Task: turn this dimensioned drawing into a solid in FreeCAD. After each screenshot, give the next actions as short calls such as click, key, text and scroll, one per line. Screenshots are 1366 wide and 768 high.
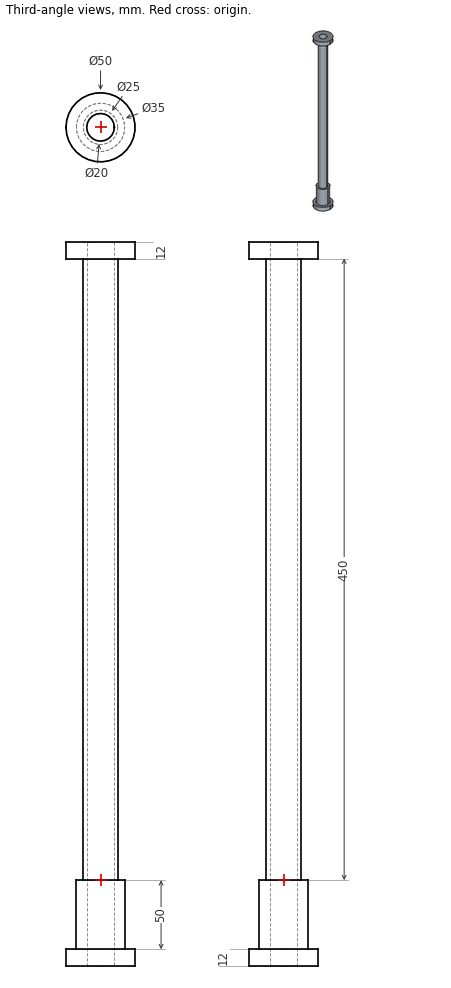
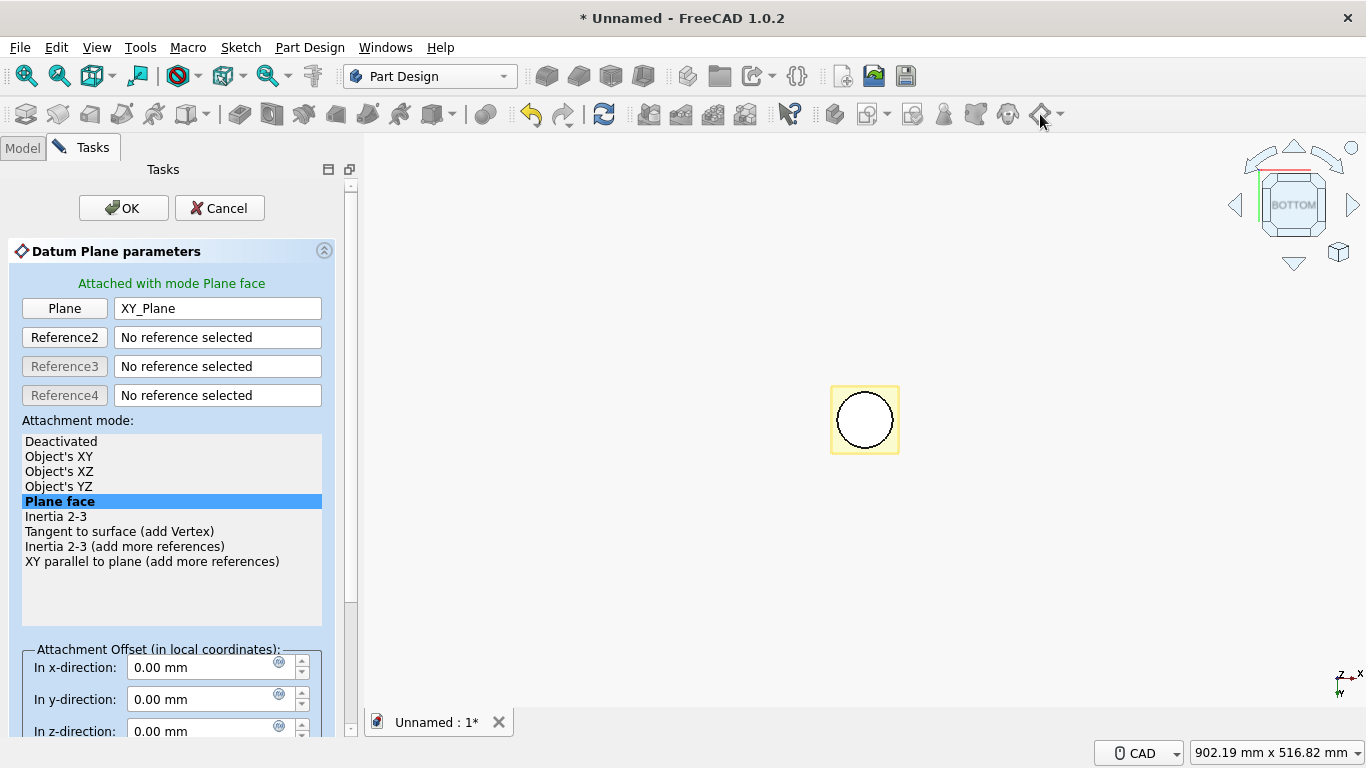
scroll(351, 458, down, 2)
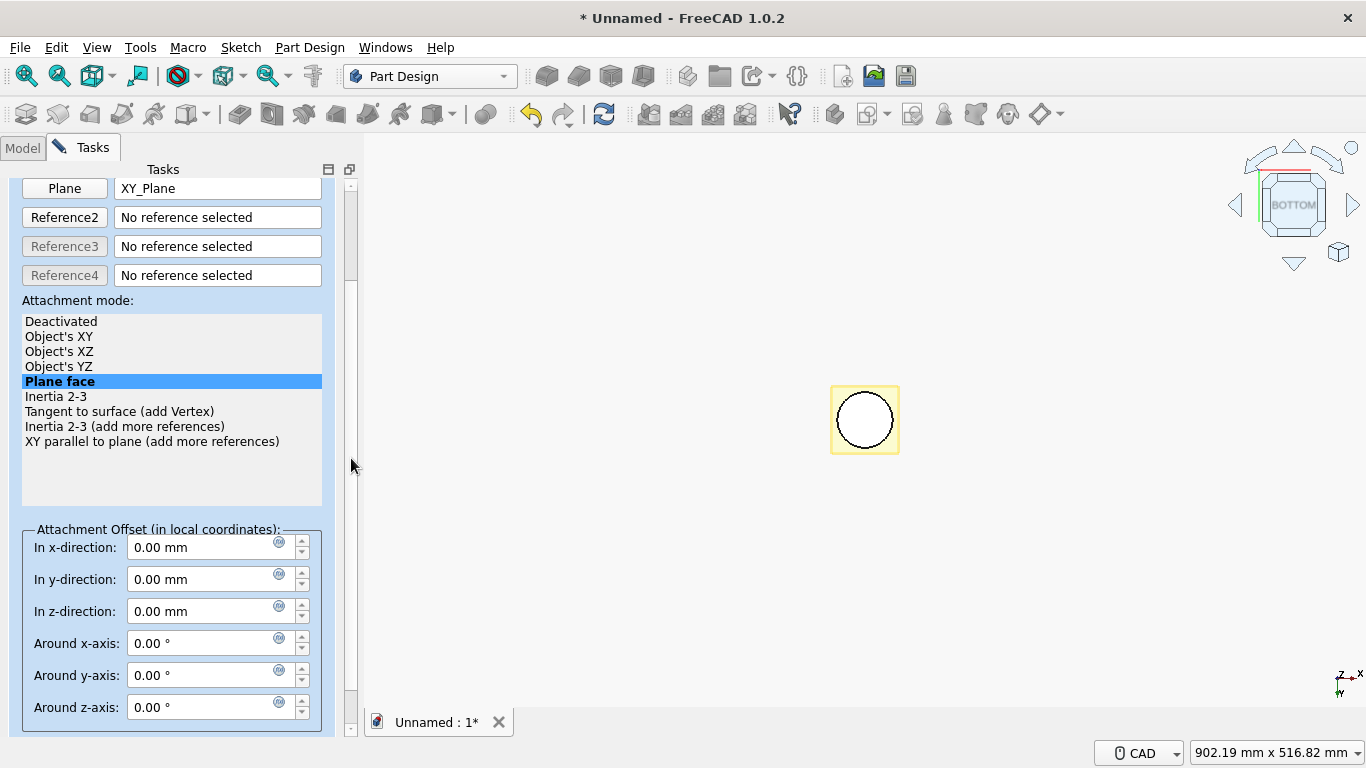
triple_click(210, 611)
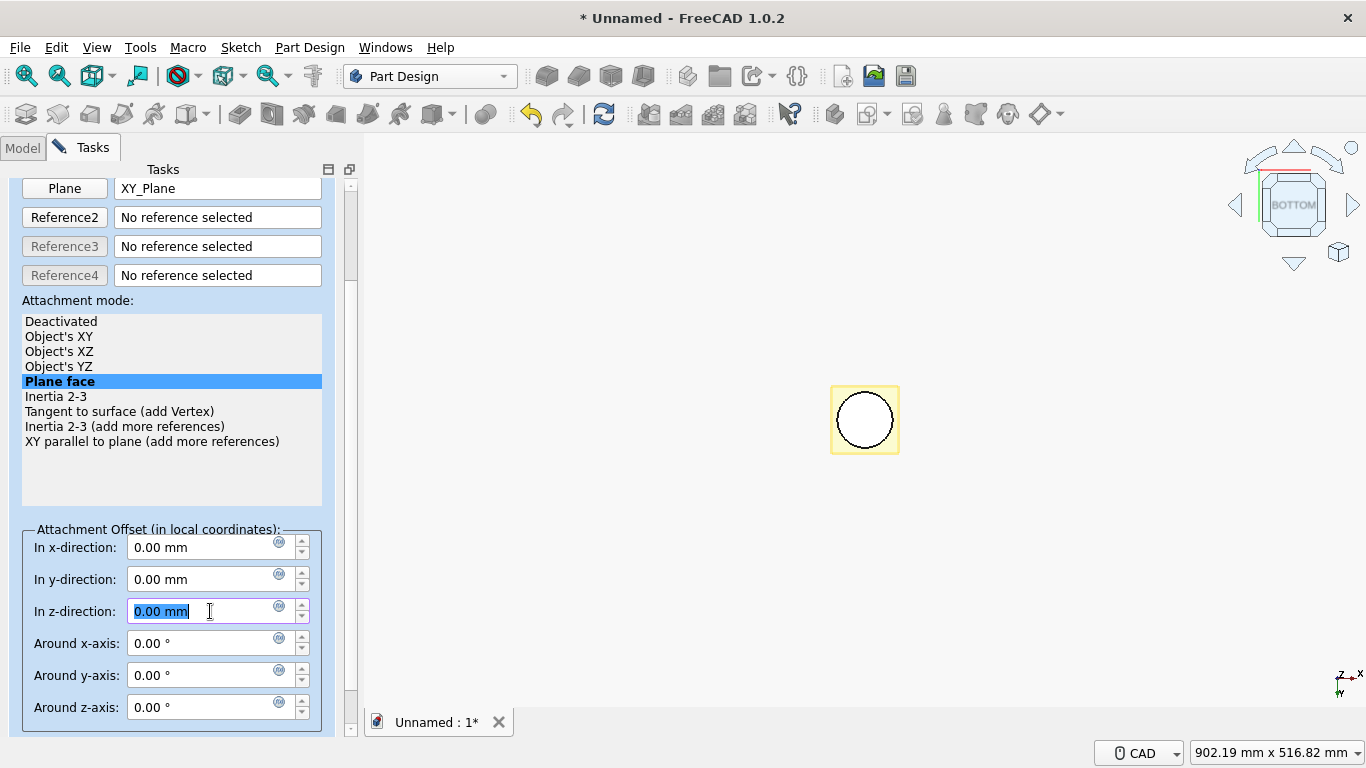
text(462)
key(Tab)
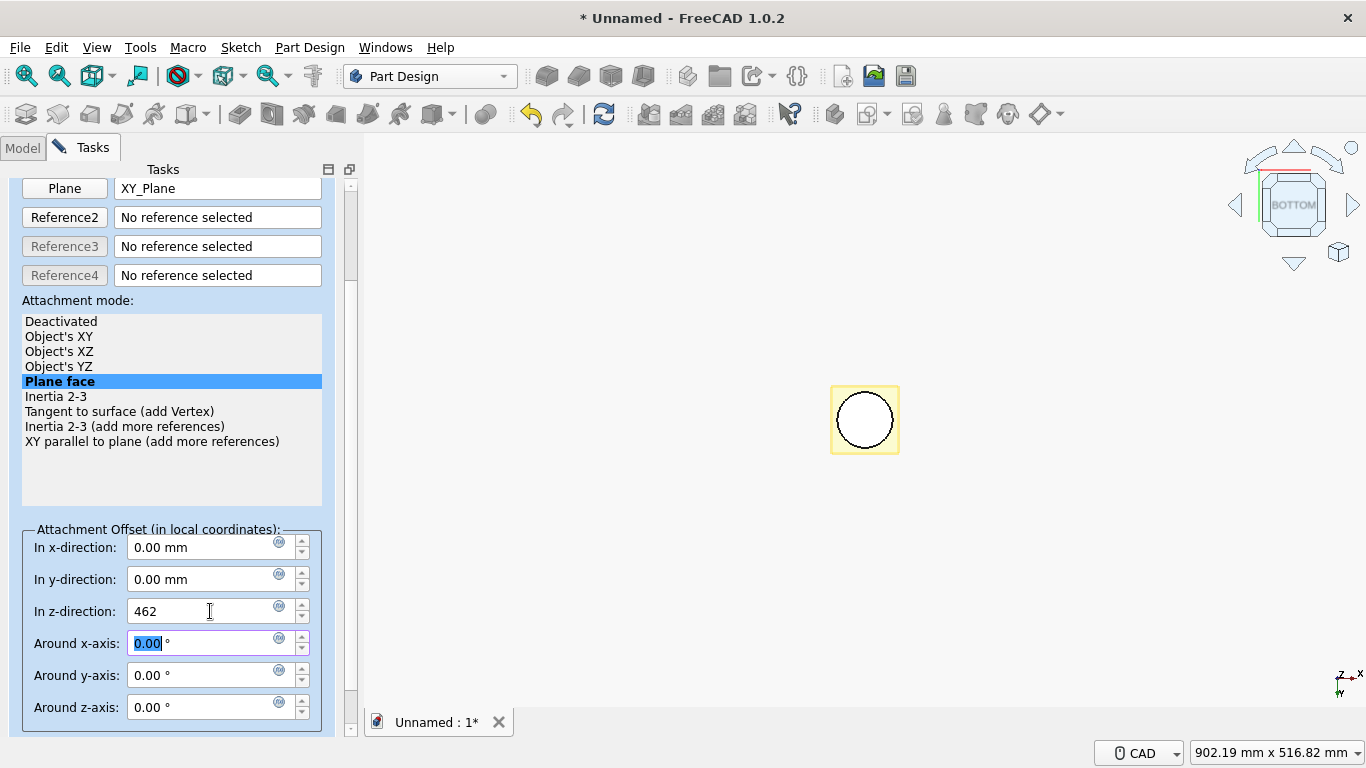
scroll(351, 458, up, 3)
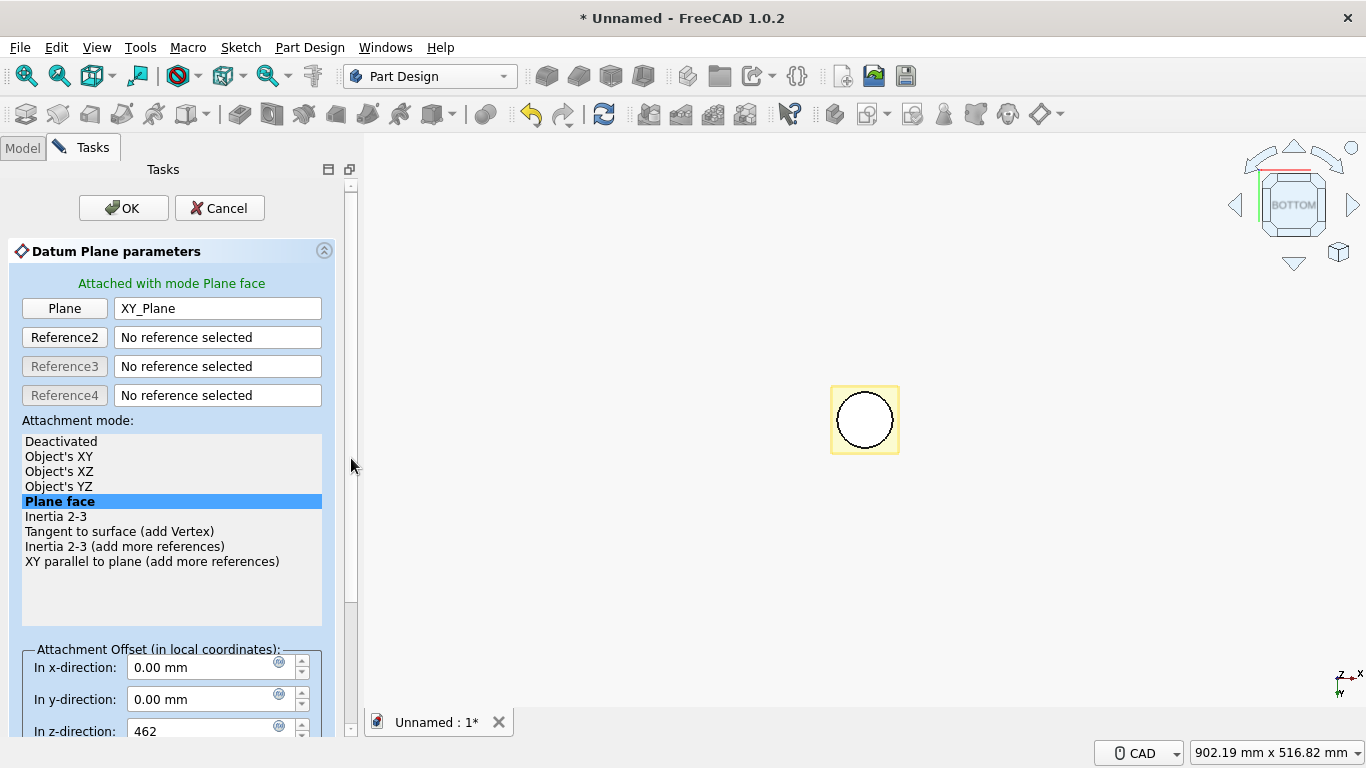
click(124, 208)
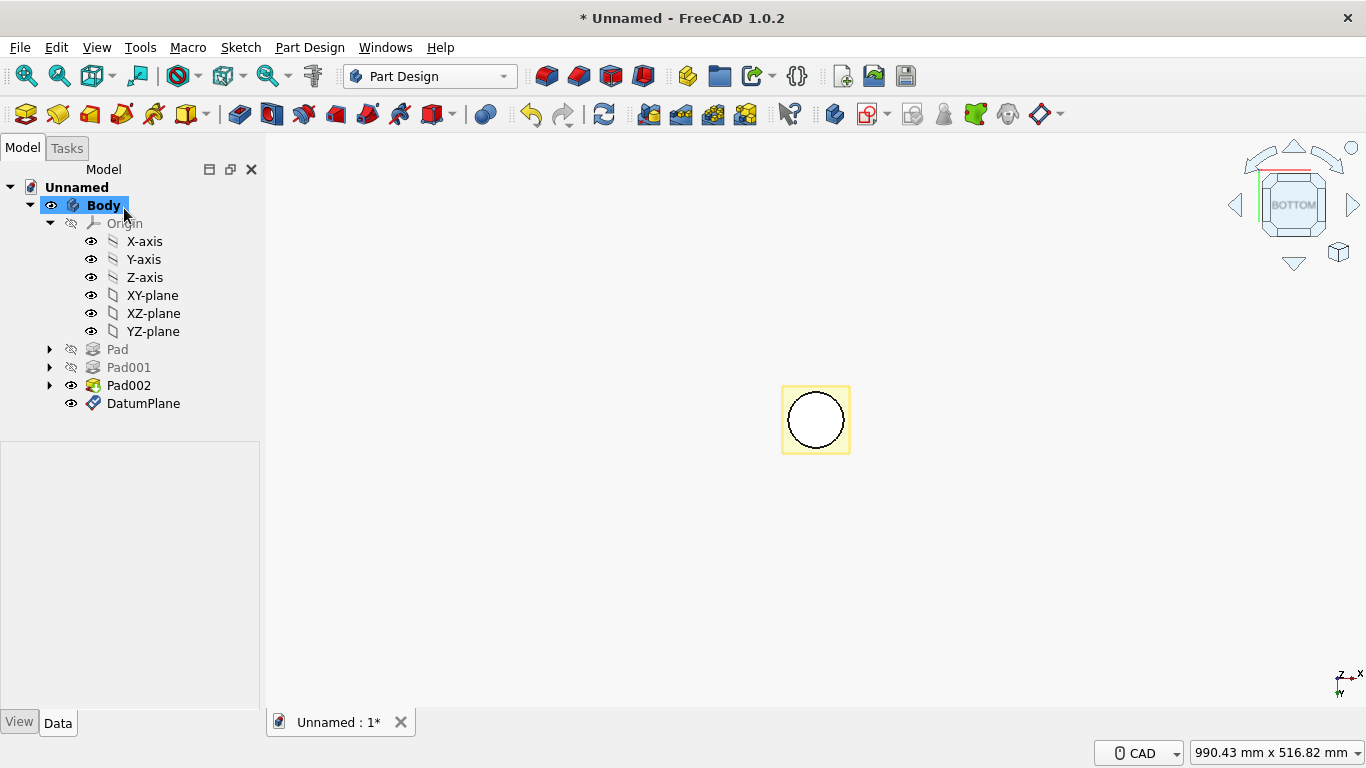
click(116, 403)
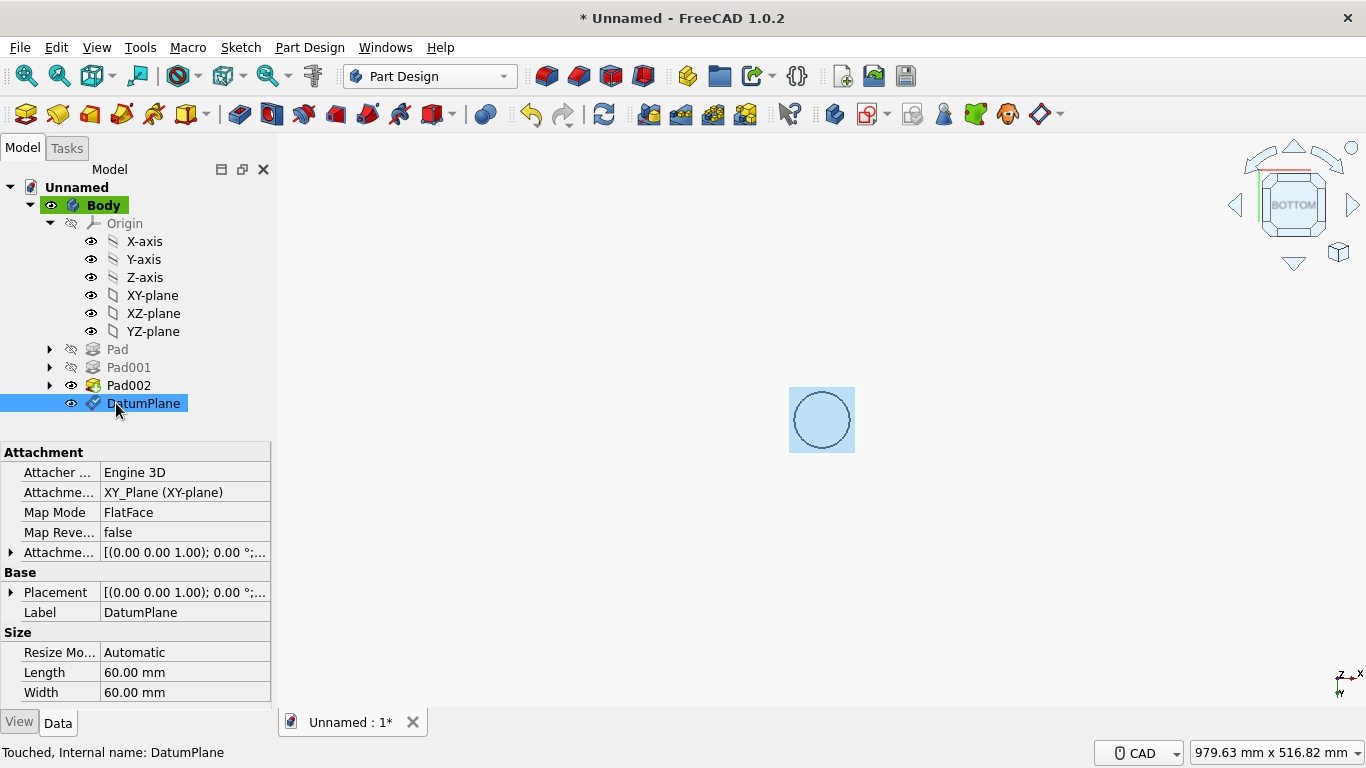
click(868, 114)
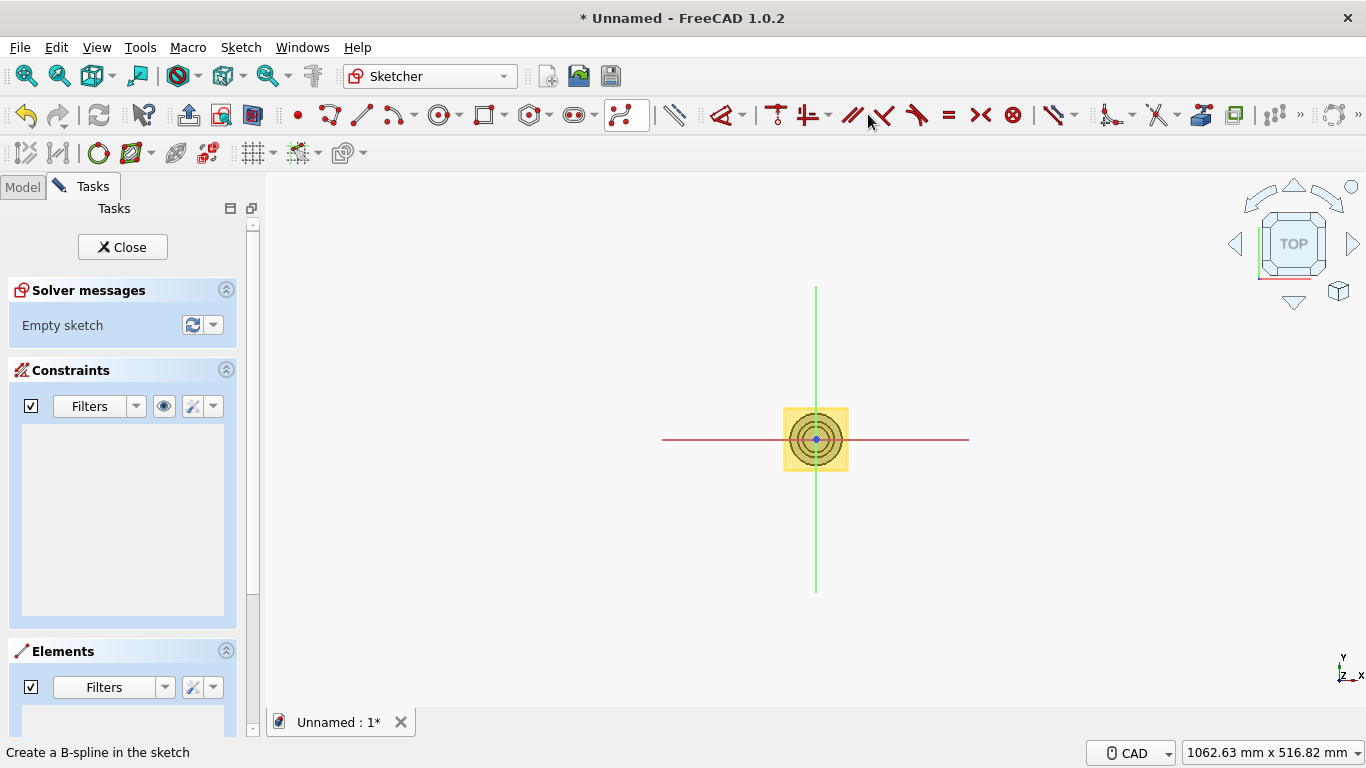
scroll(830, 440, up, 9)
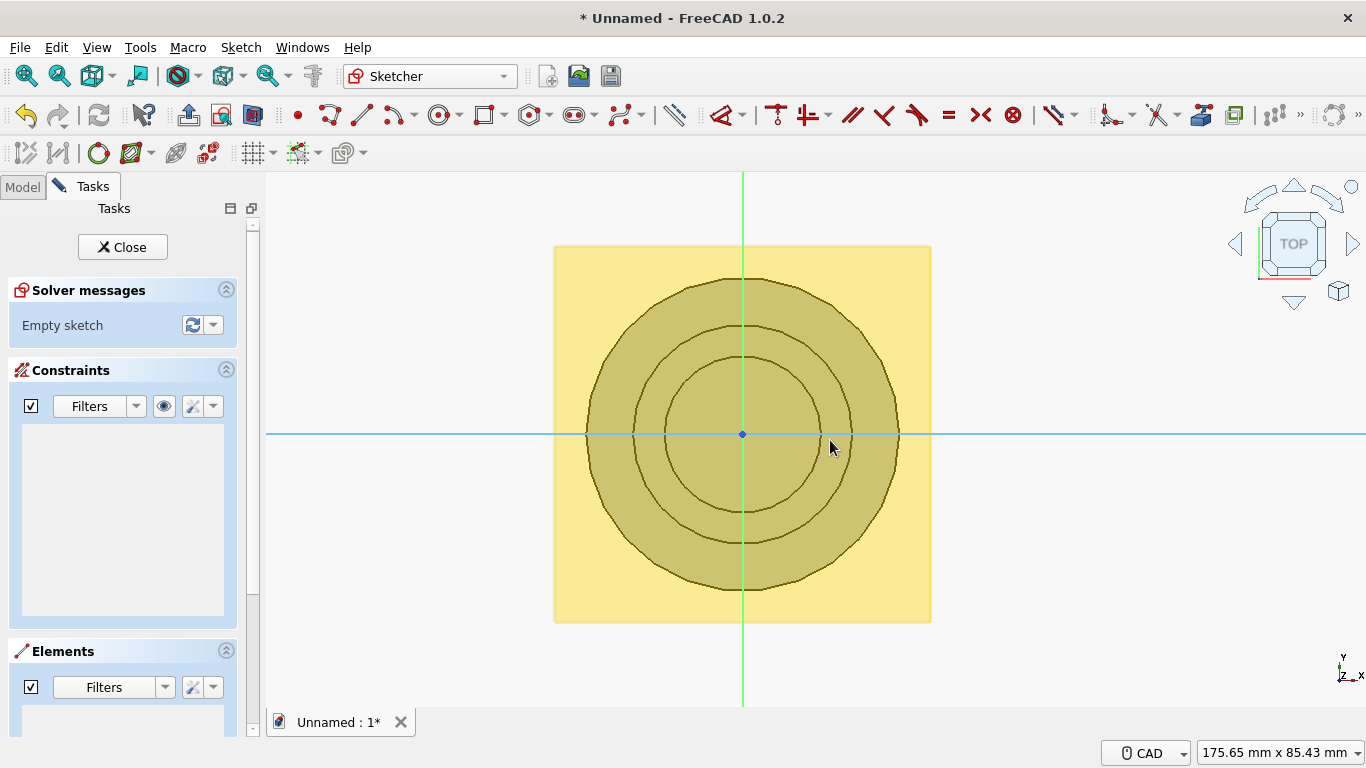
click(440, 116)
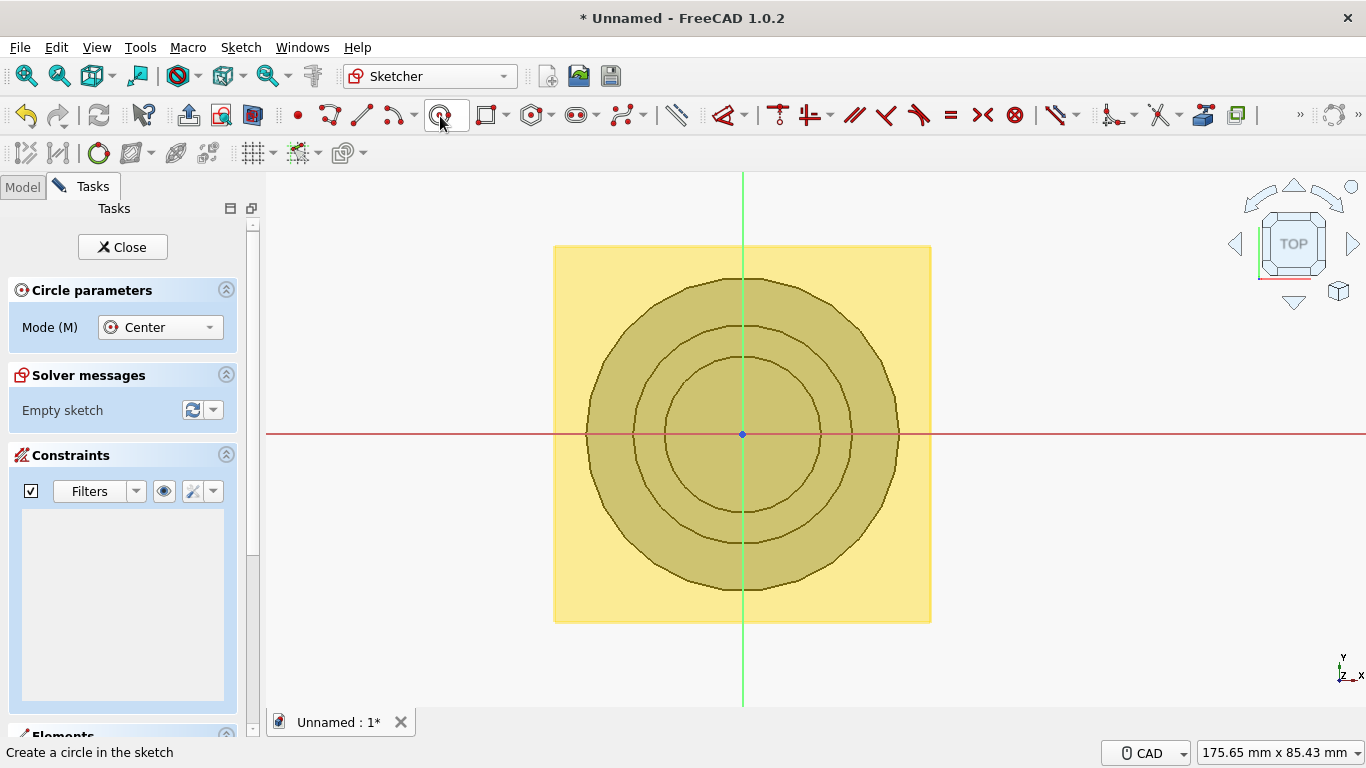
click(743, 434)
click(853, 324)
key(Escape)